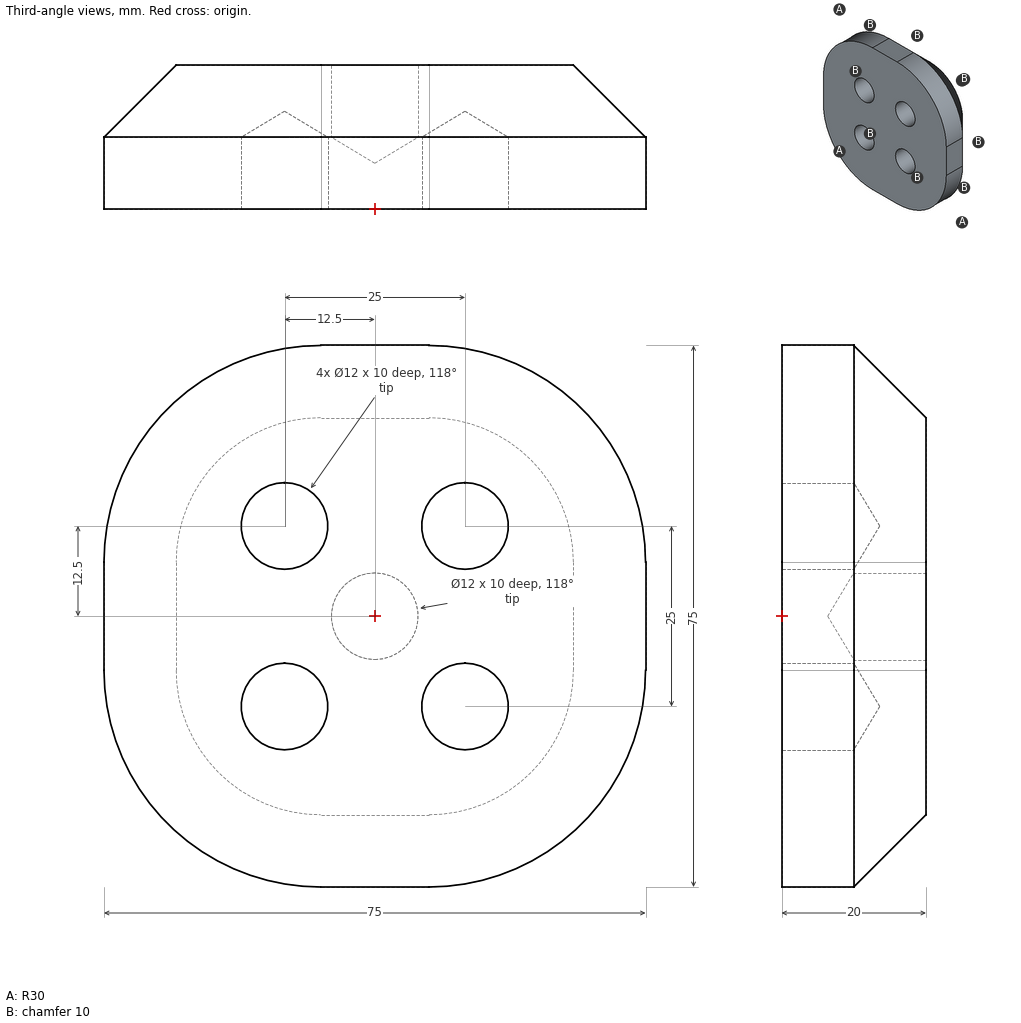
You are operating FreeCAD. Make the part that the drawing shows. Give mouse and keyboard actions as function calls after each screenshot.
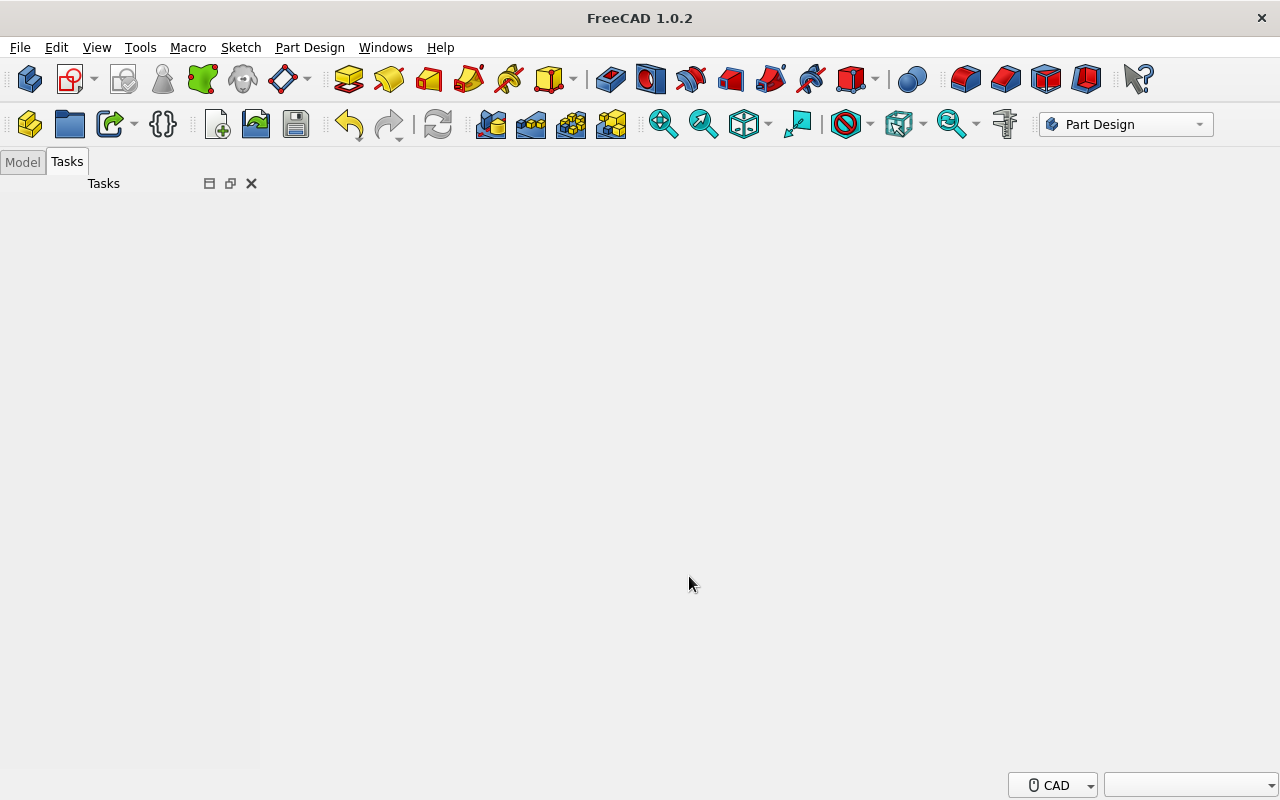
click(216, 124)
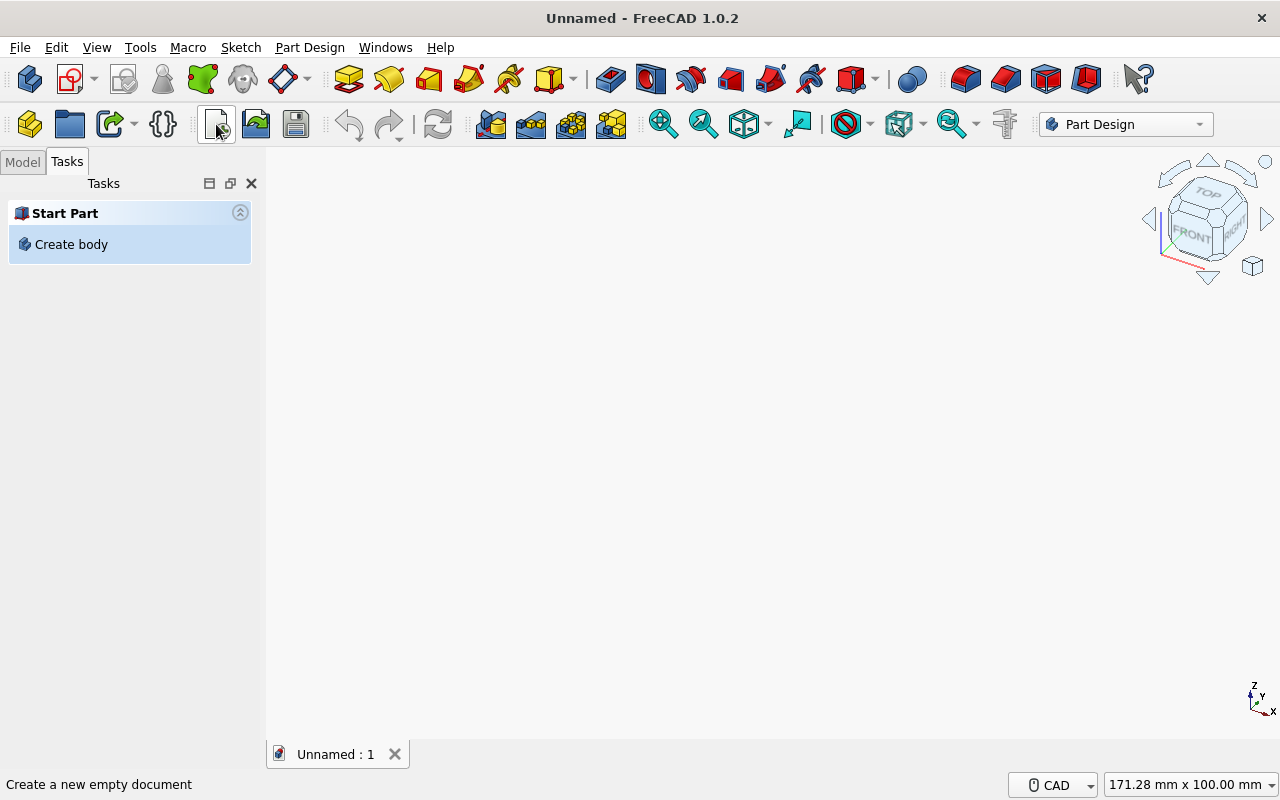
click(70, 80)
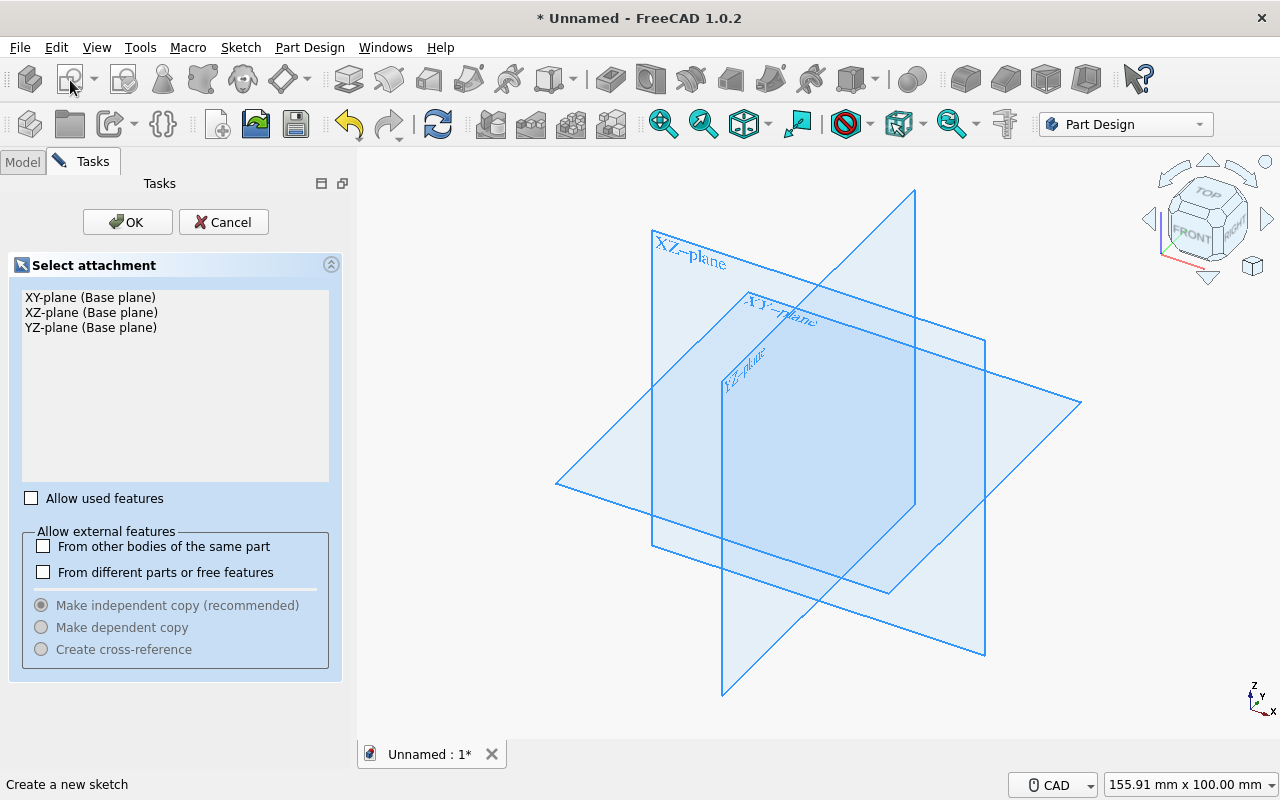
click(82, 312)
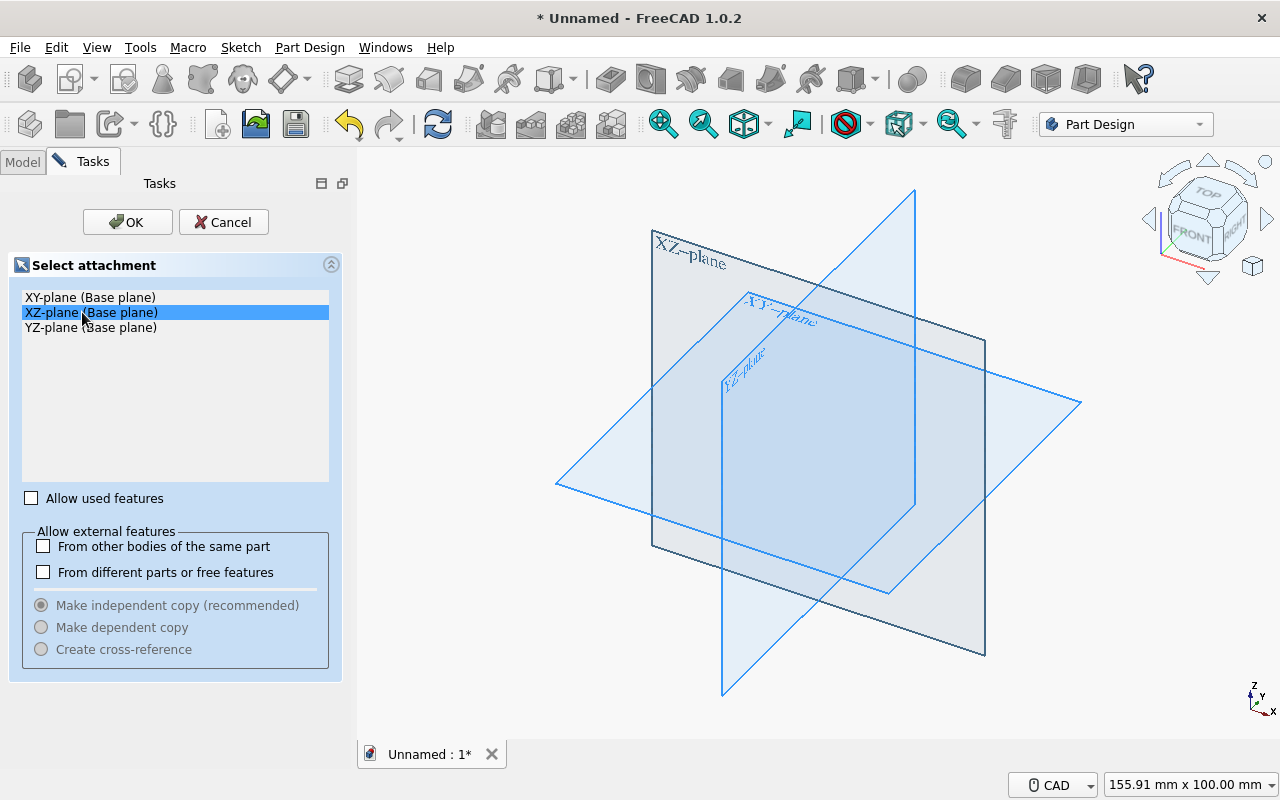
click(128, 222)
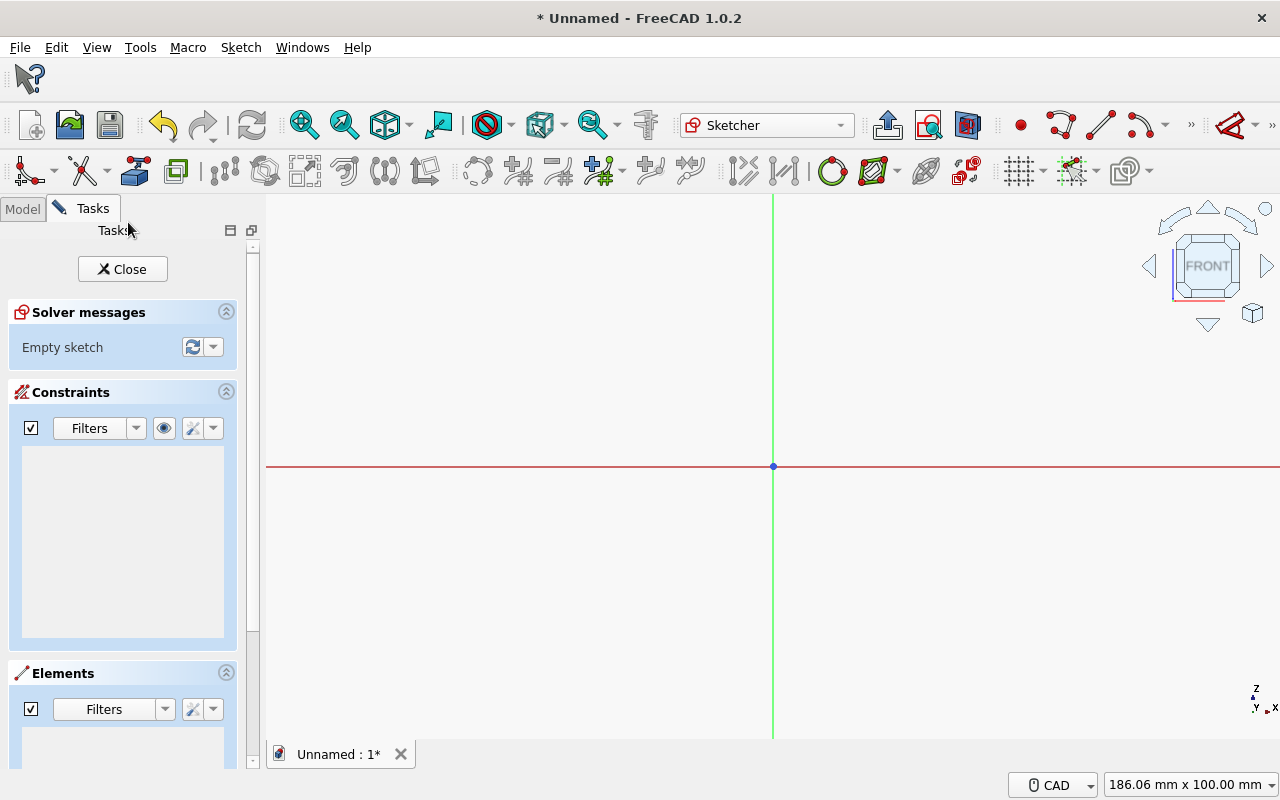
key(g)
key(v)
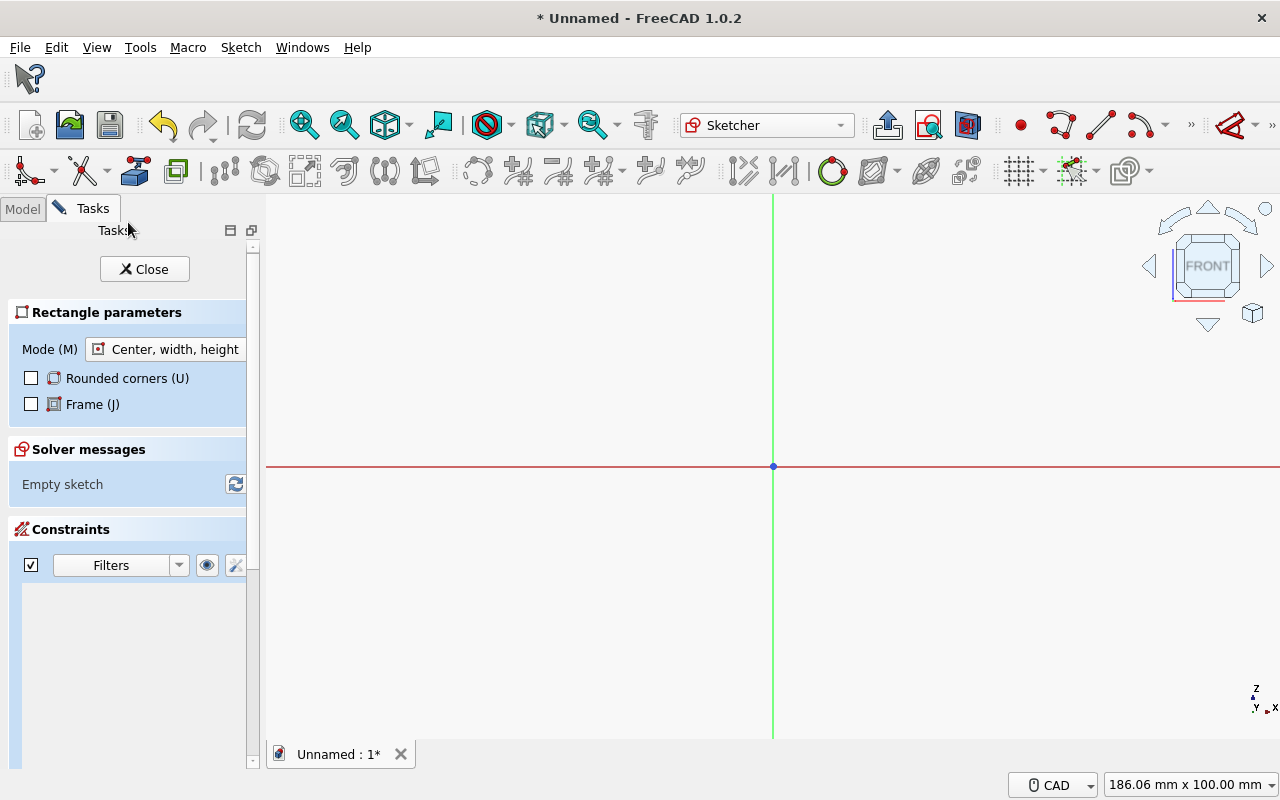
click(773, 466)
click(977, 262)
key(Escape)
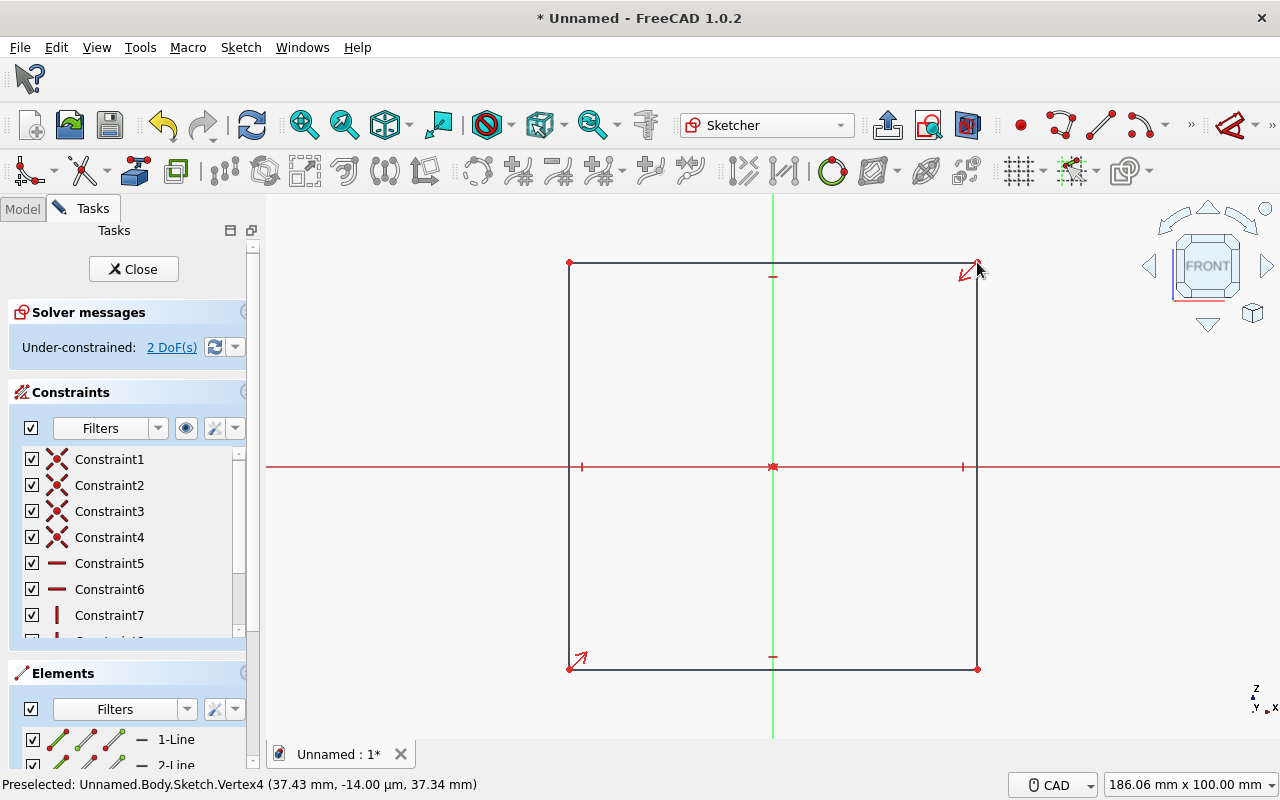
key(d)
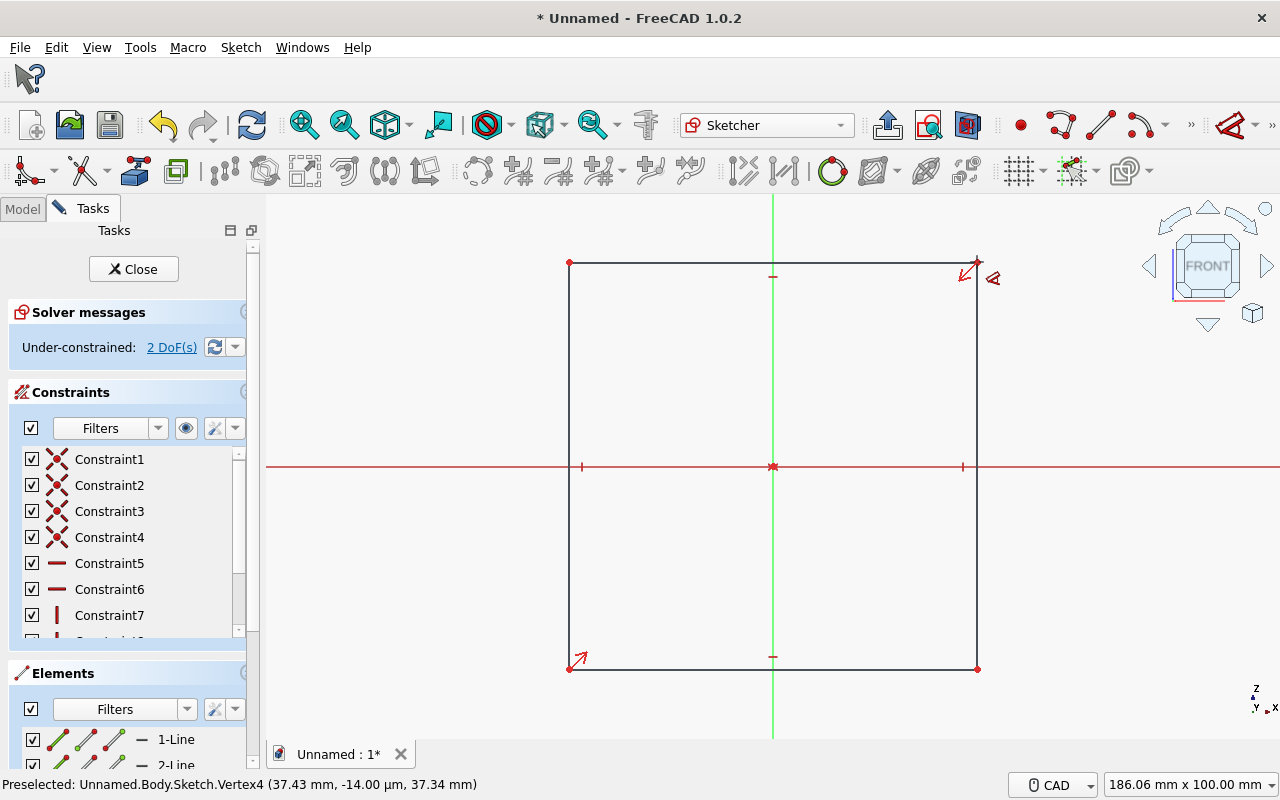
click(691, 670)
click(679, 704)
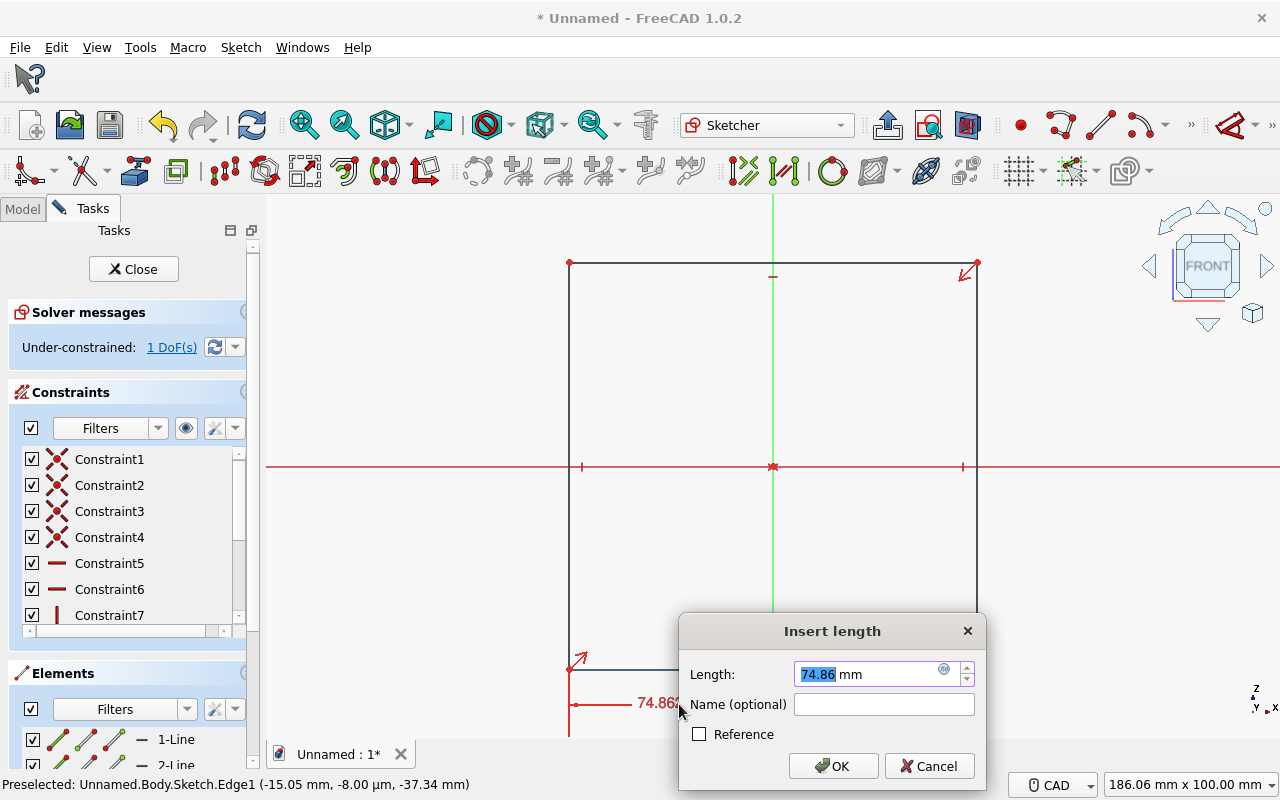
text(75)
key(Return)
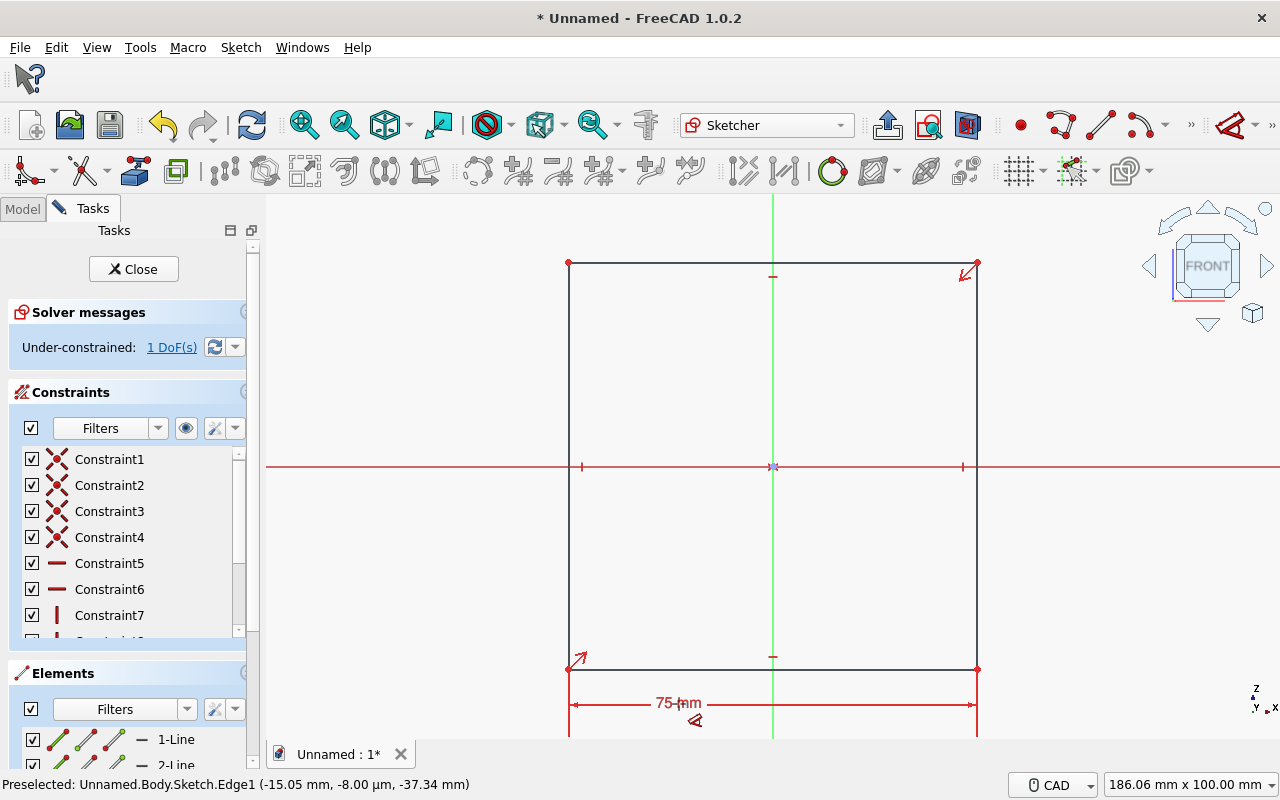
click(977, 548)
click(1011, 373)